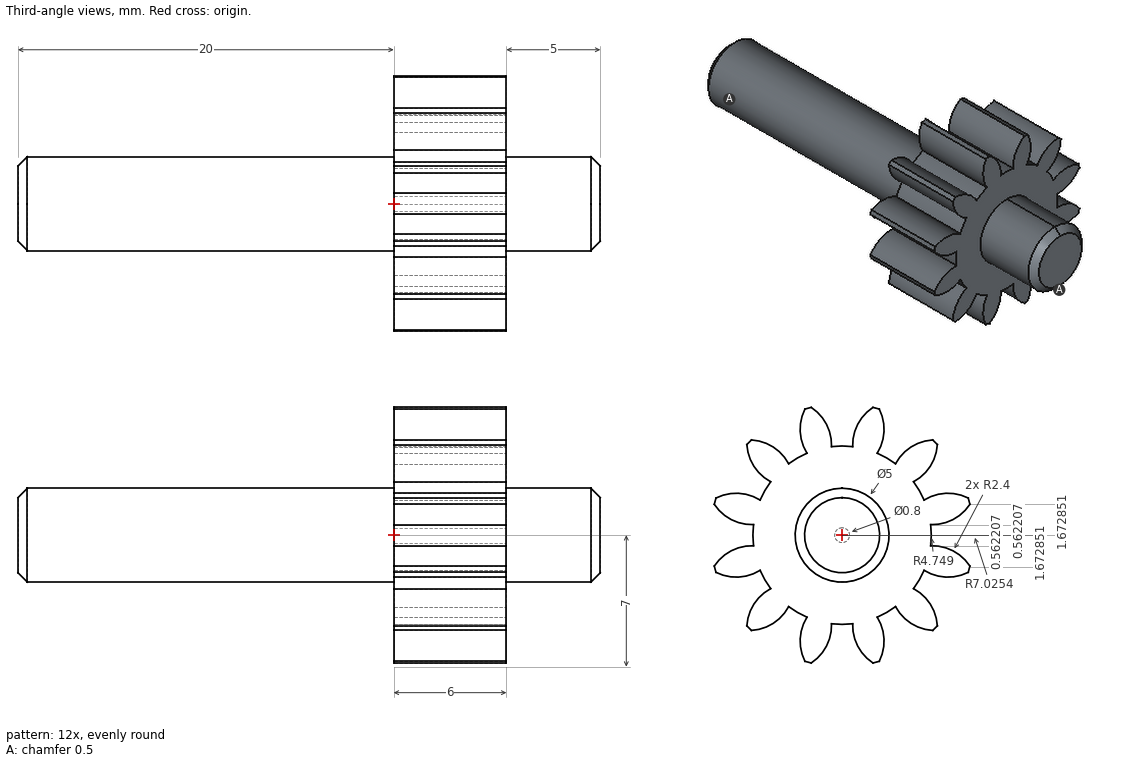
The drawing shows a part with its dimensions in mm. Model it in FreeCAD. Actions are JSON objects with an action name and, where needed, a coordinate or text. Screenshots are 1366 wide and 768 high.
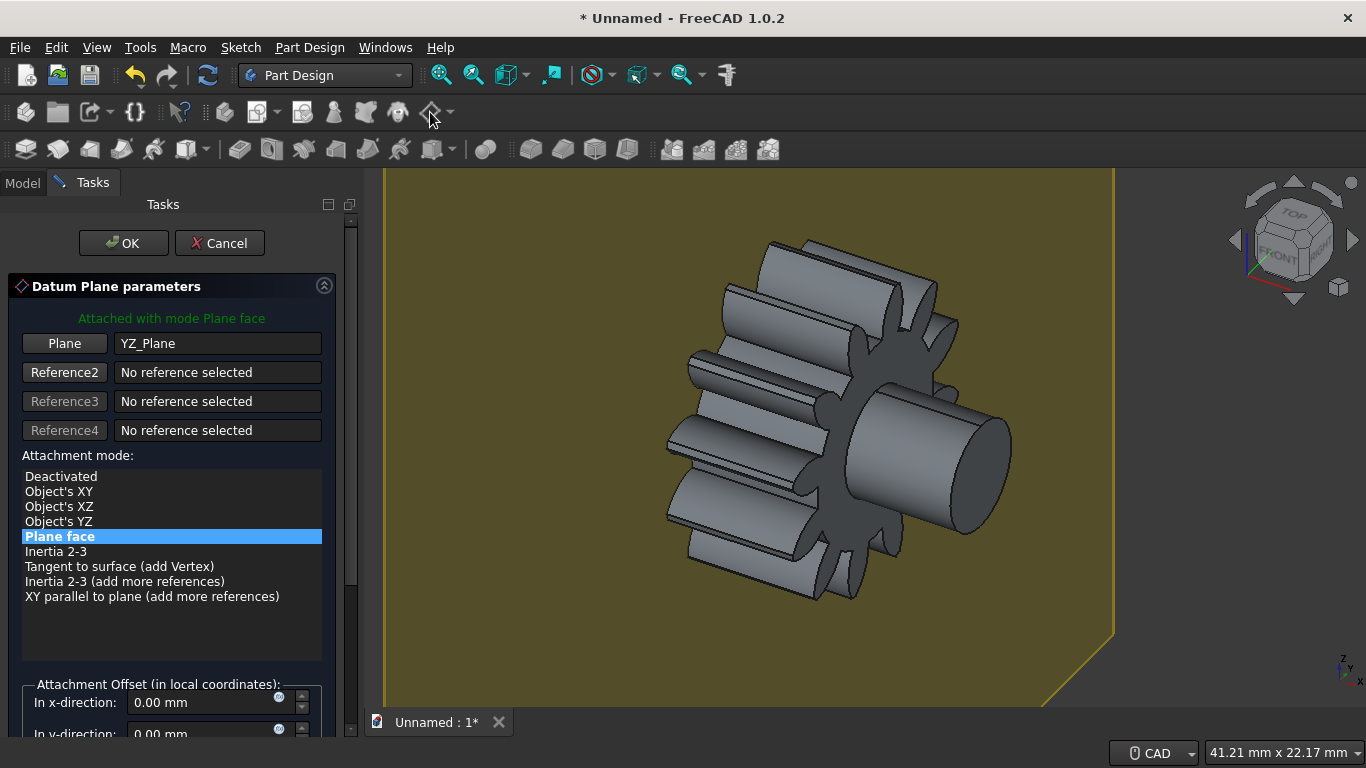
{"action": "scroll", "coordinate": [351, 475], "scroll_direction": "down", "scroll_amount": 2}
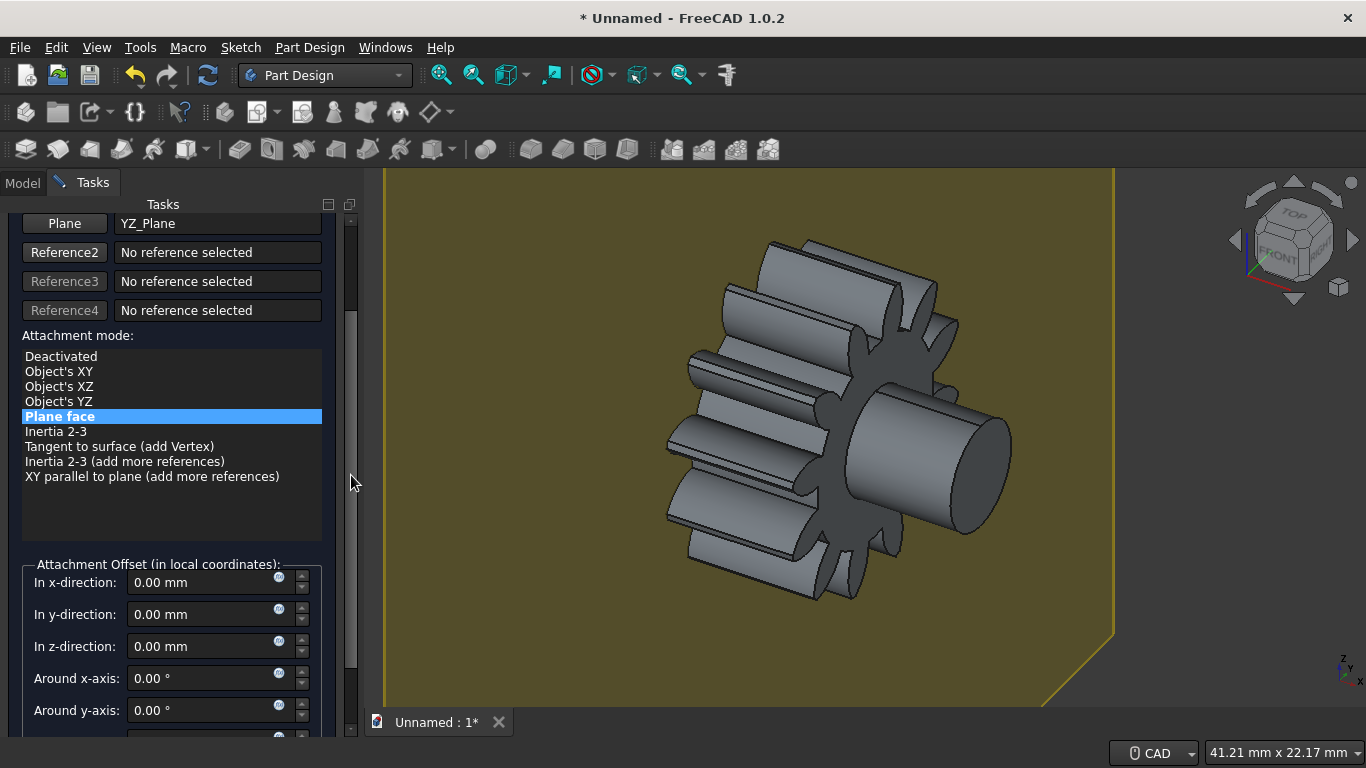
{"action": "triple_click", "coordinate": [210, 646]}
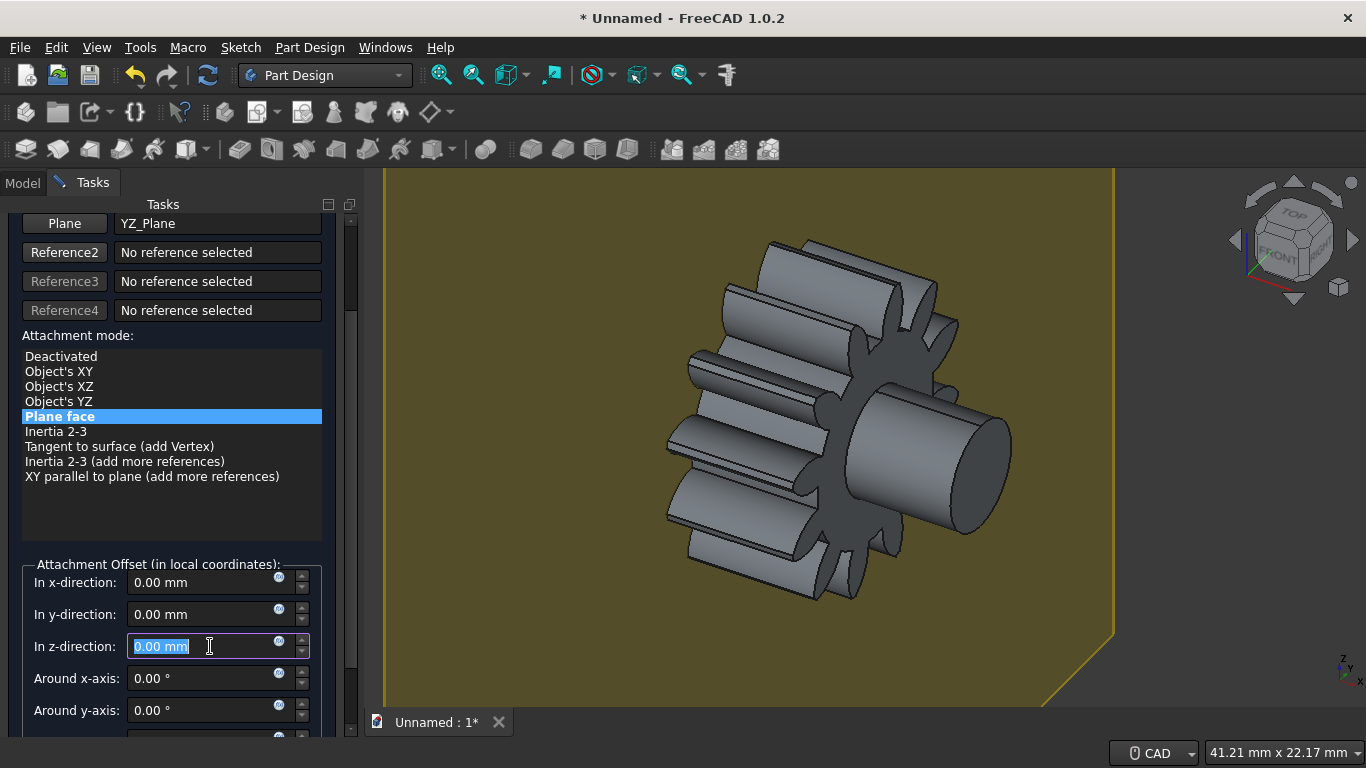
{"action": "type", "text": "-20"}
{"action": "key", "text": "Tab"}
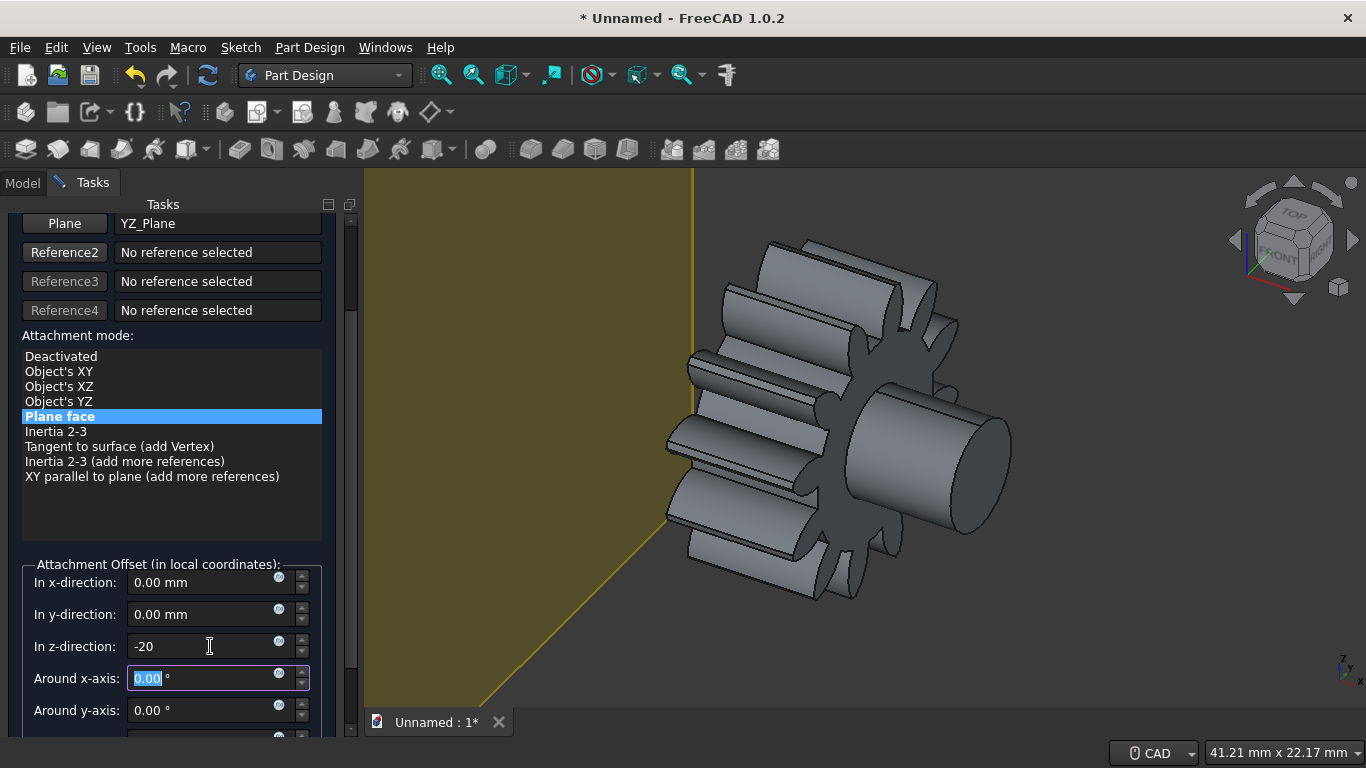
{"action": "scroll", "coordinate": [351, 475], "scroll_direction": "up", "scroll_amount": 3}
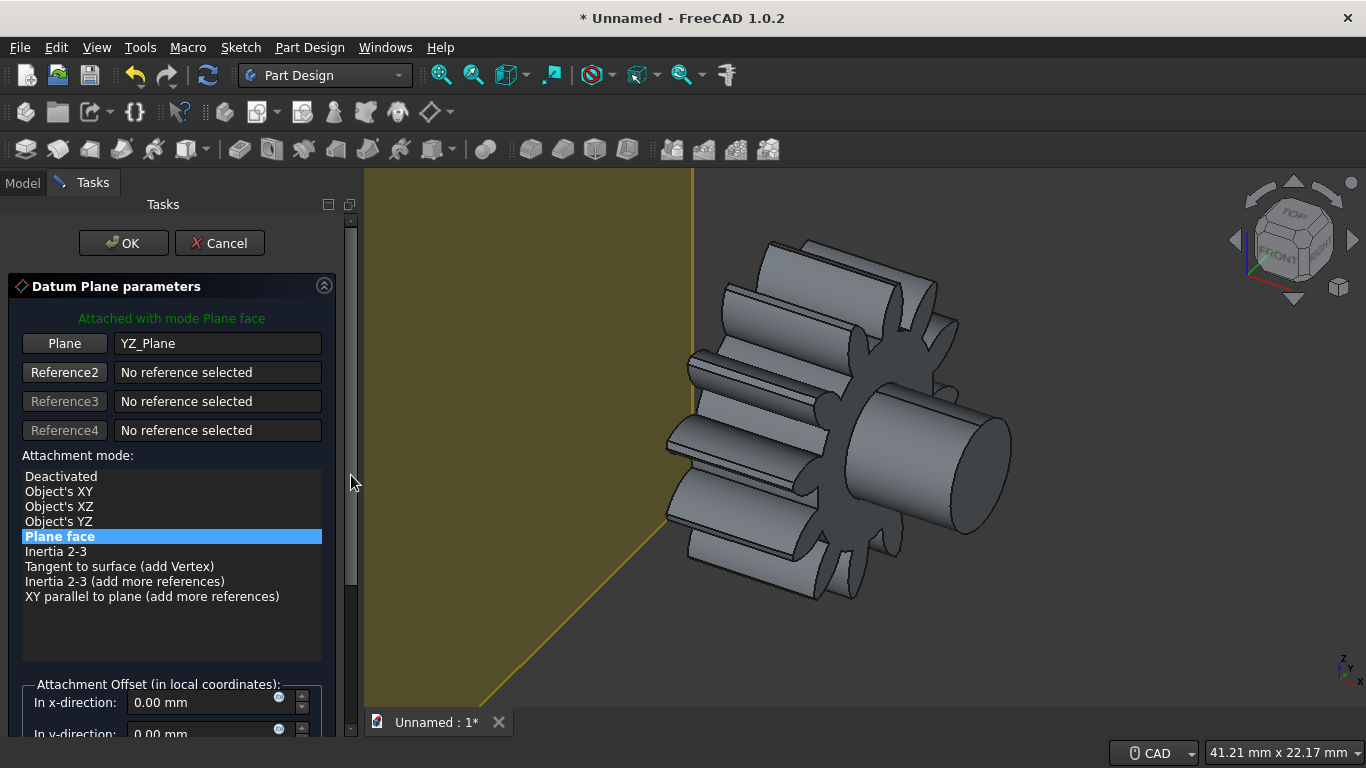
{"action": "left_click", "coordinate": [124, 243]}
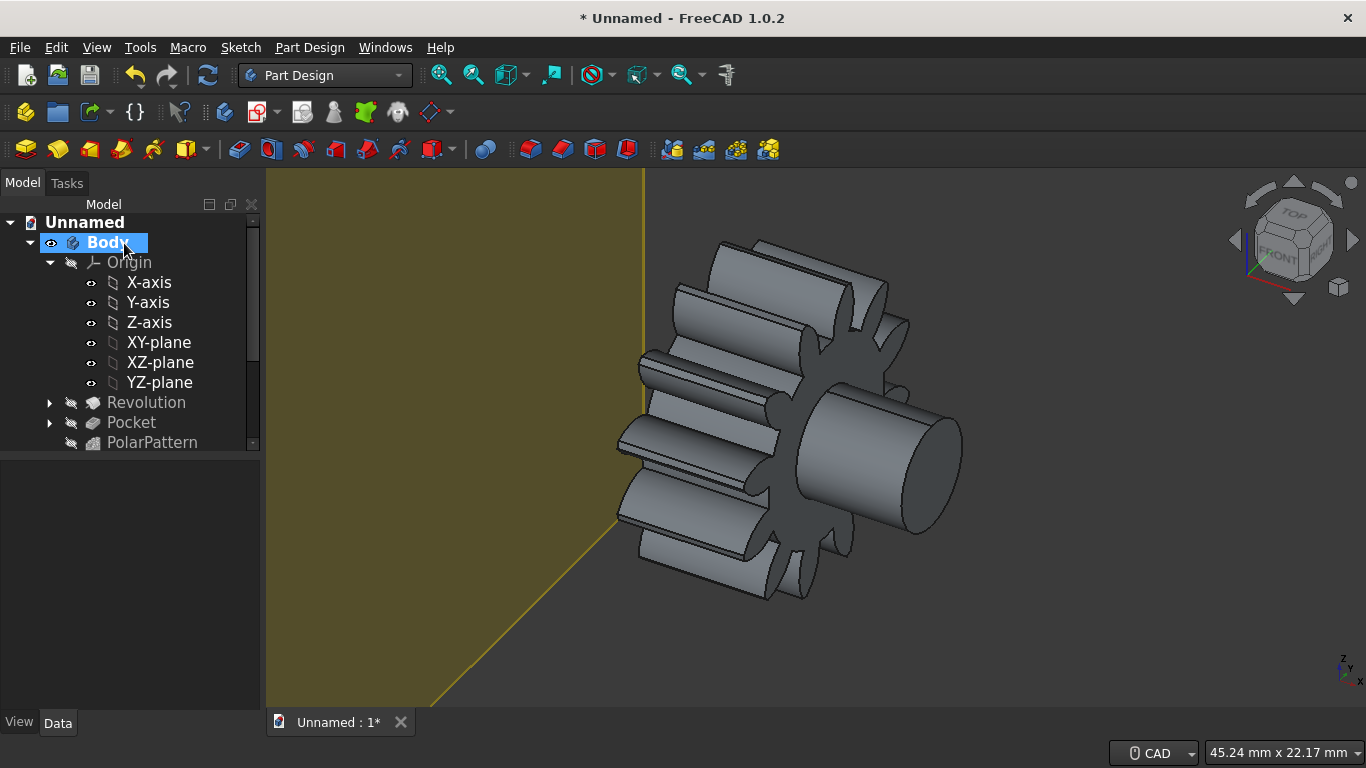
{"action": "scroll", "coordinate": [100, 338], "scroll_direction": "down", "scroll_amount": 3}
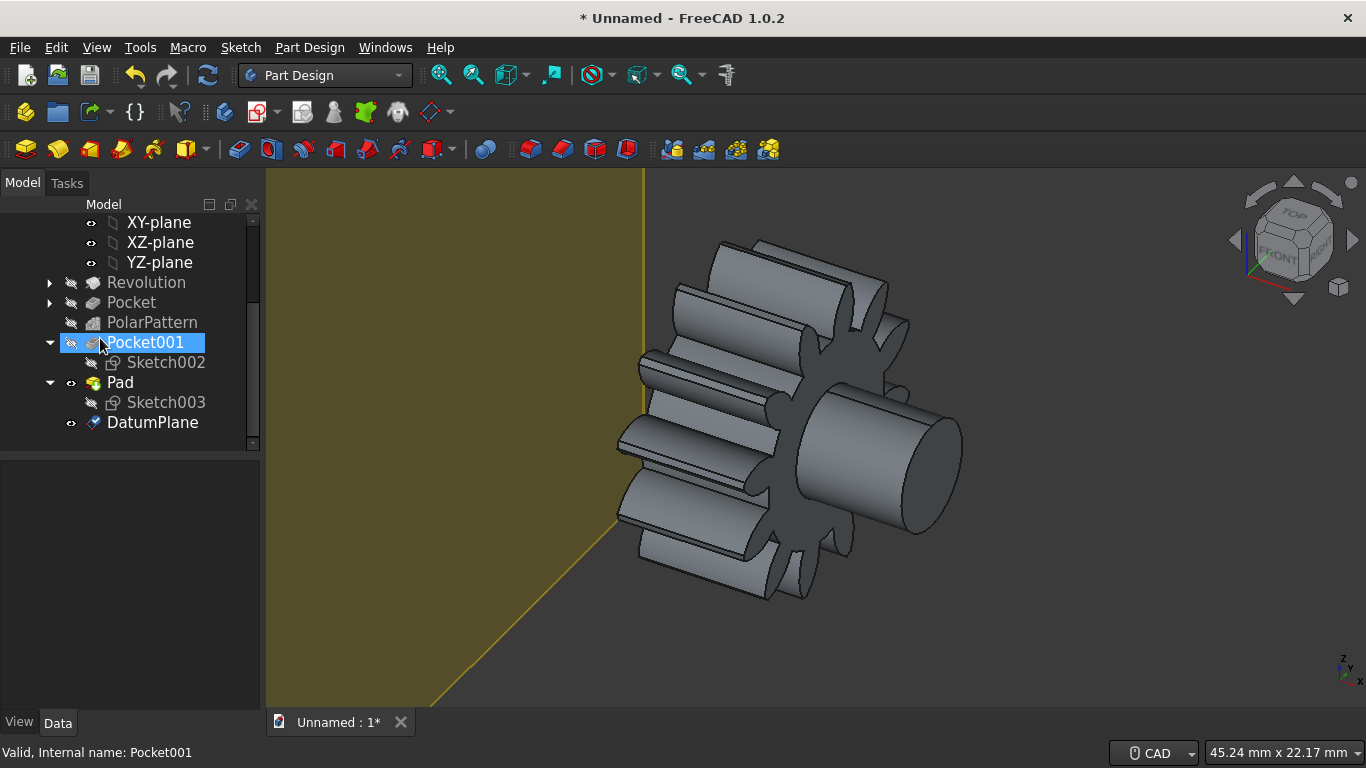
{"action": "left_click", "coordinate": [116, 423]}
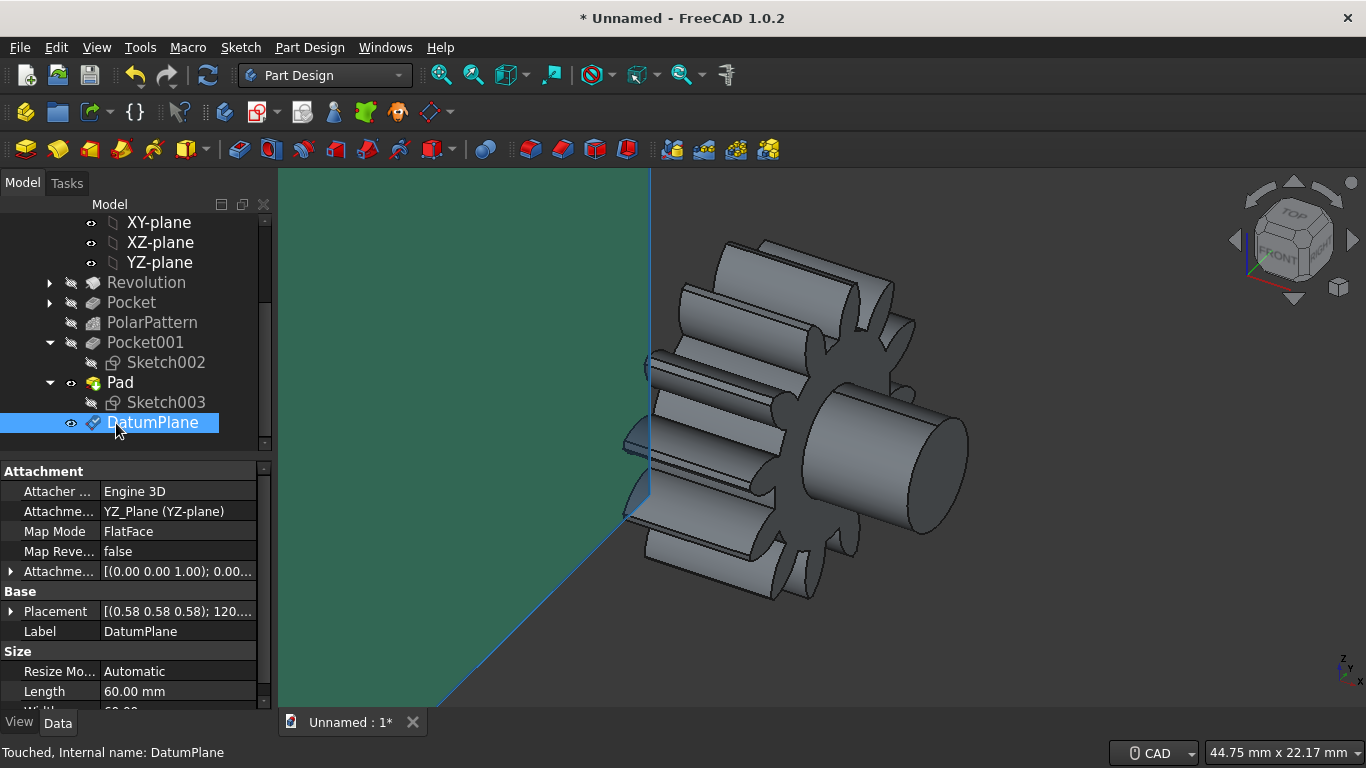
{"action": "left_click", "coordinate": [258, 112]}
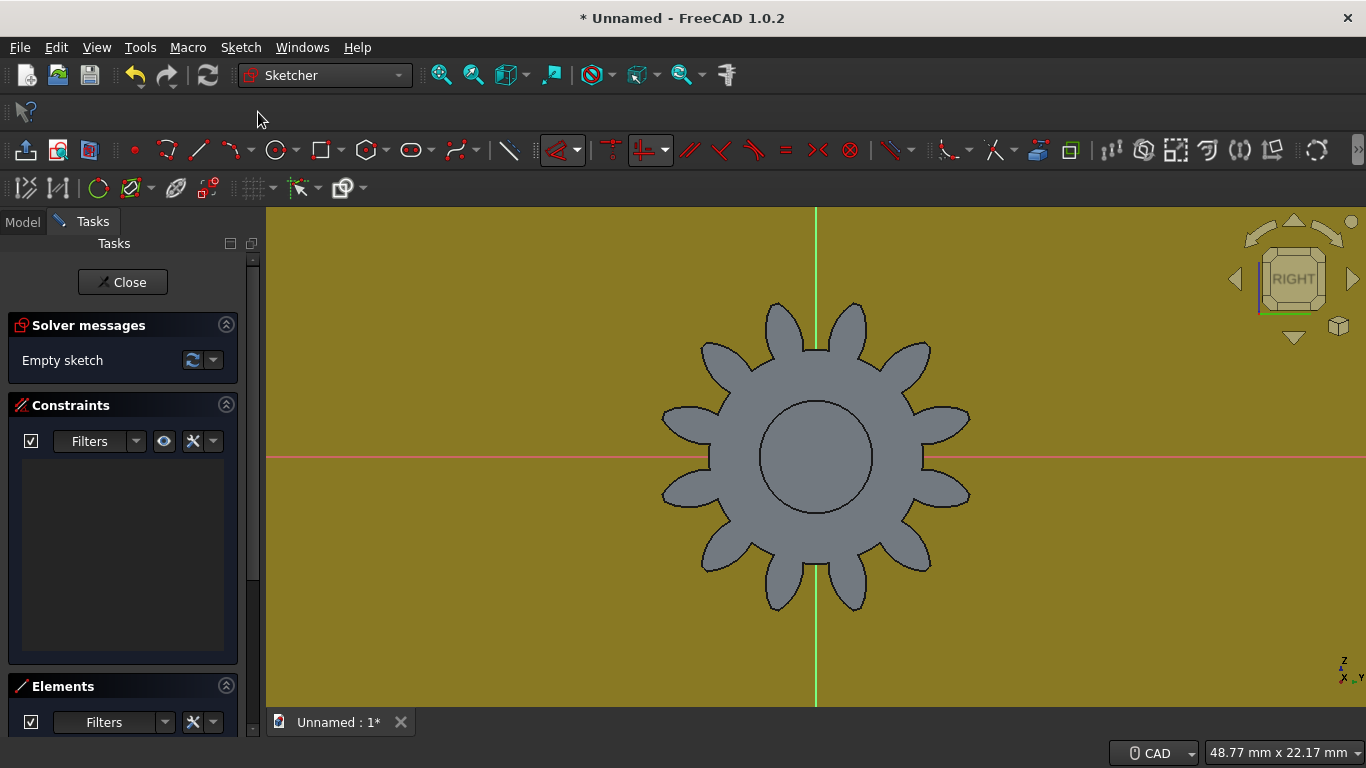
{"action": "key", "text": "q s"}